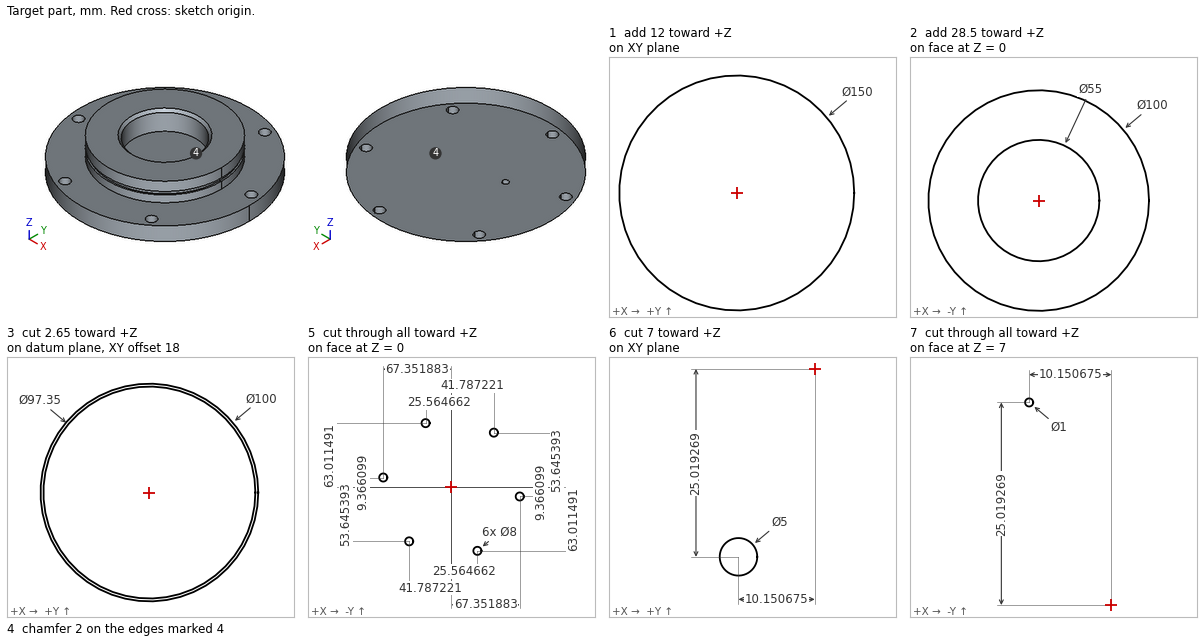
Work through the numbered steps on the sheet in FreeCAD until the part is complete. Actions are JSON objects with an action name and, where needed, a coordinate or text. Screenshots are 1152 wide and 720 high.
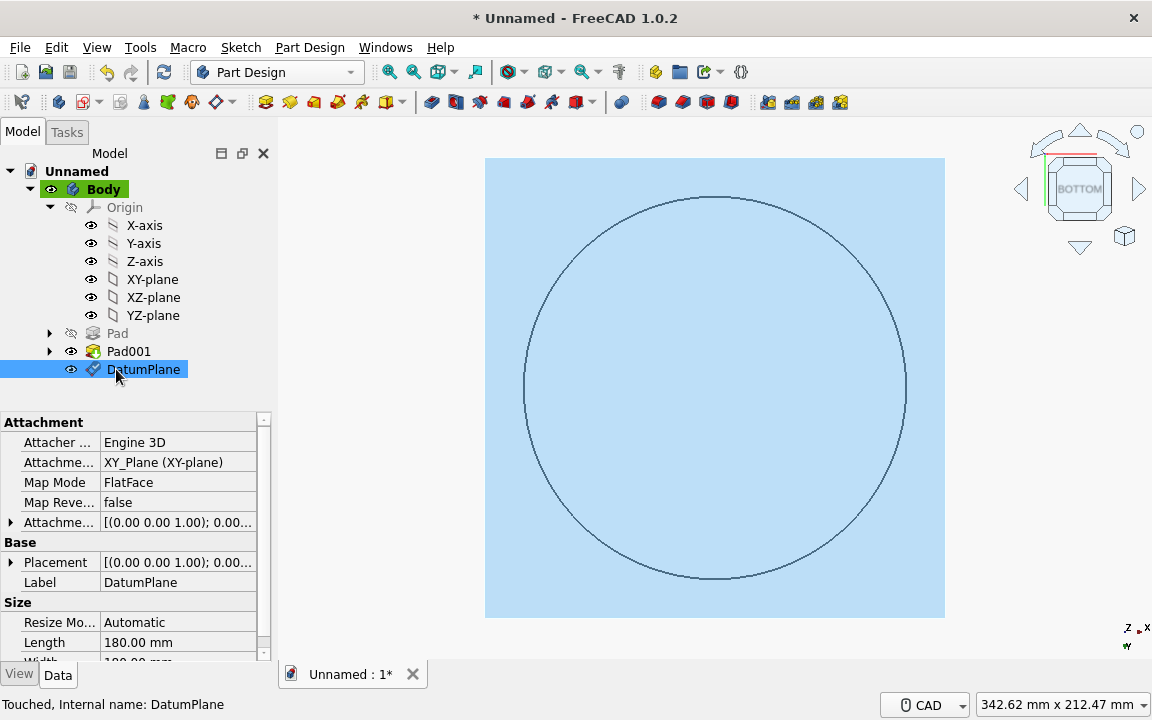
{"action": "left_click", "coordinate": [84, 102]}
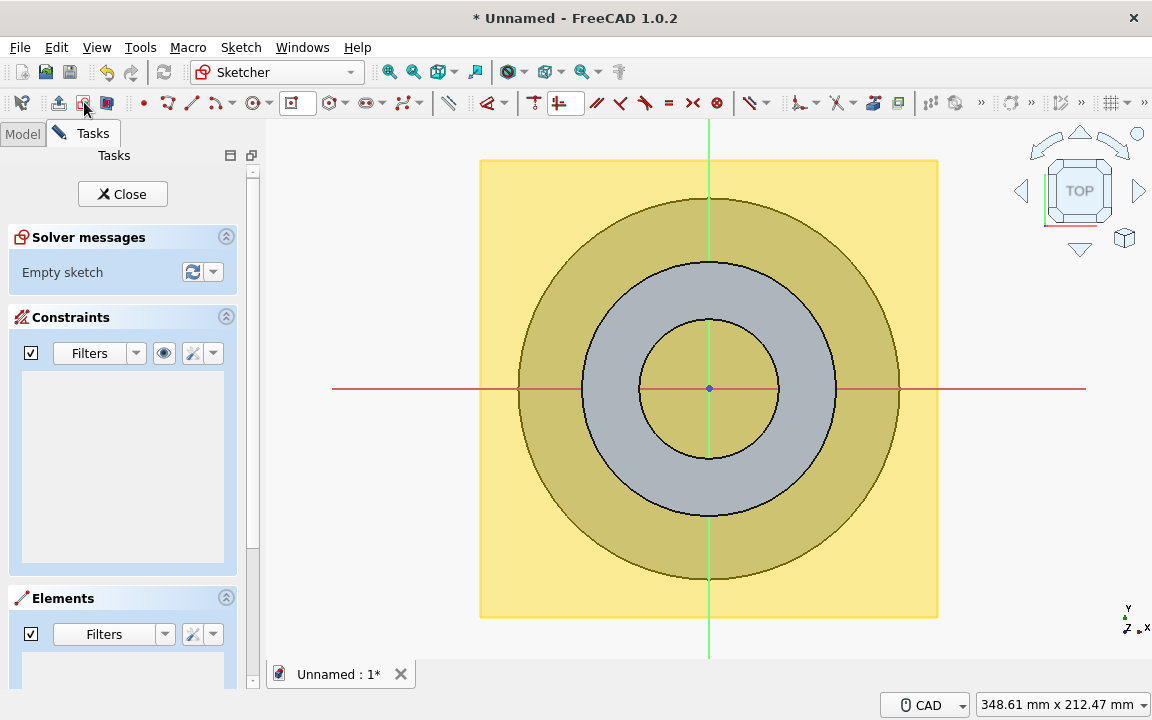
{"action": "key", "text": "q s"}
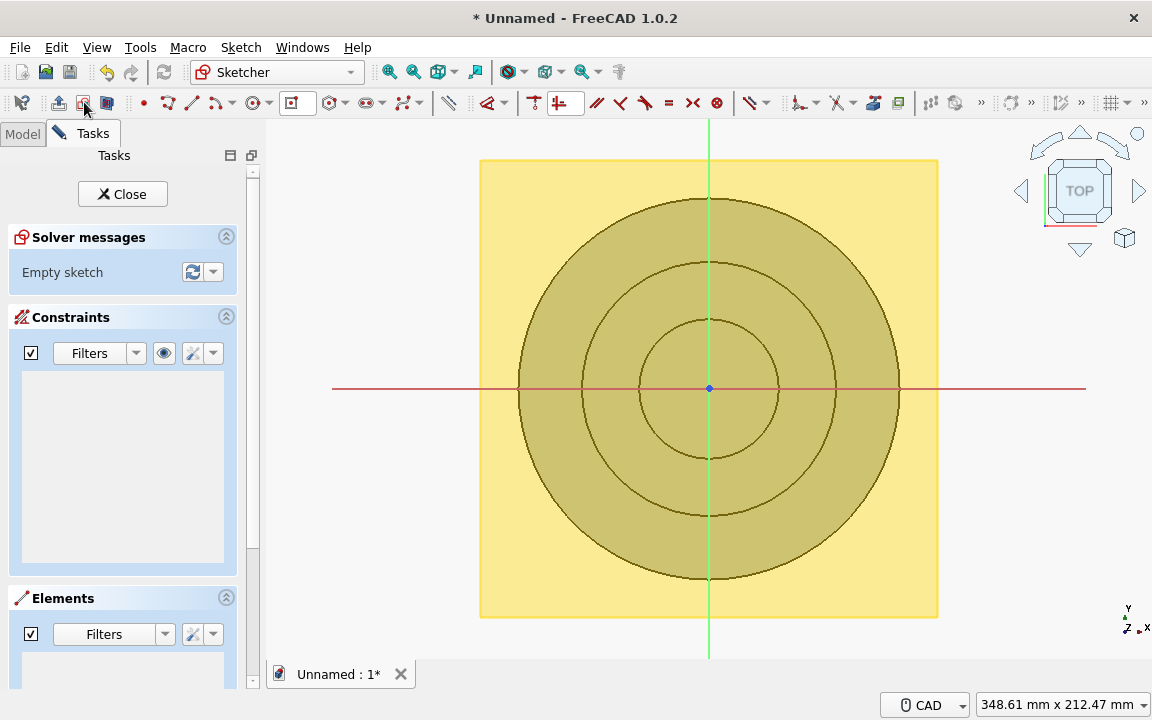
{"action": "left_click", "coordinate": [254, 104]}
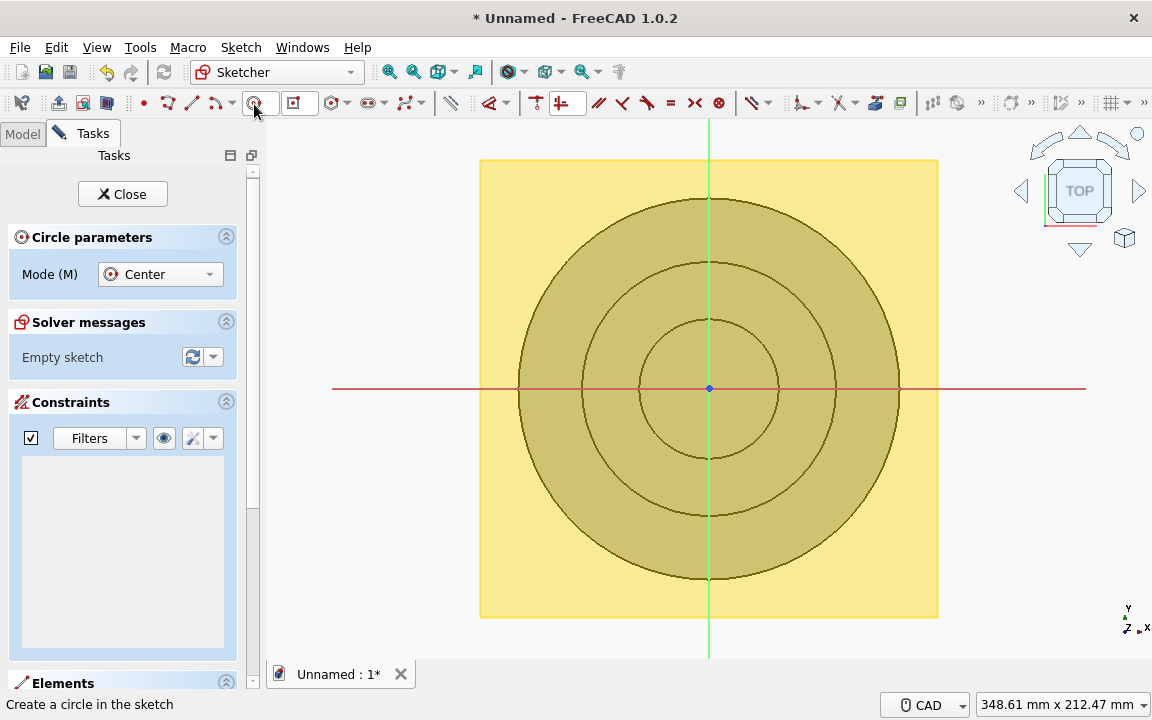
{"action": "left_click", "coordinate": [709, 389]}
{"action": "mouse_move", "coordinate": [799, 299]}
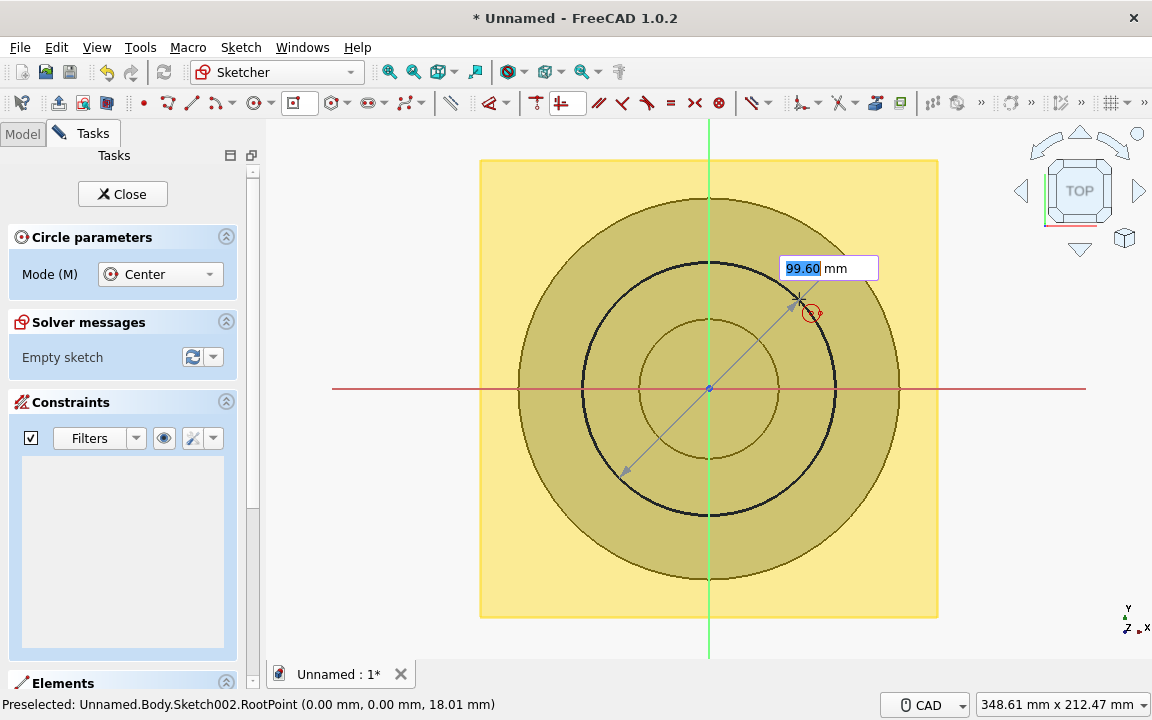
{"action": "type", "text": "100"}
{"action": "key", "text": "Return"}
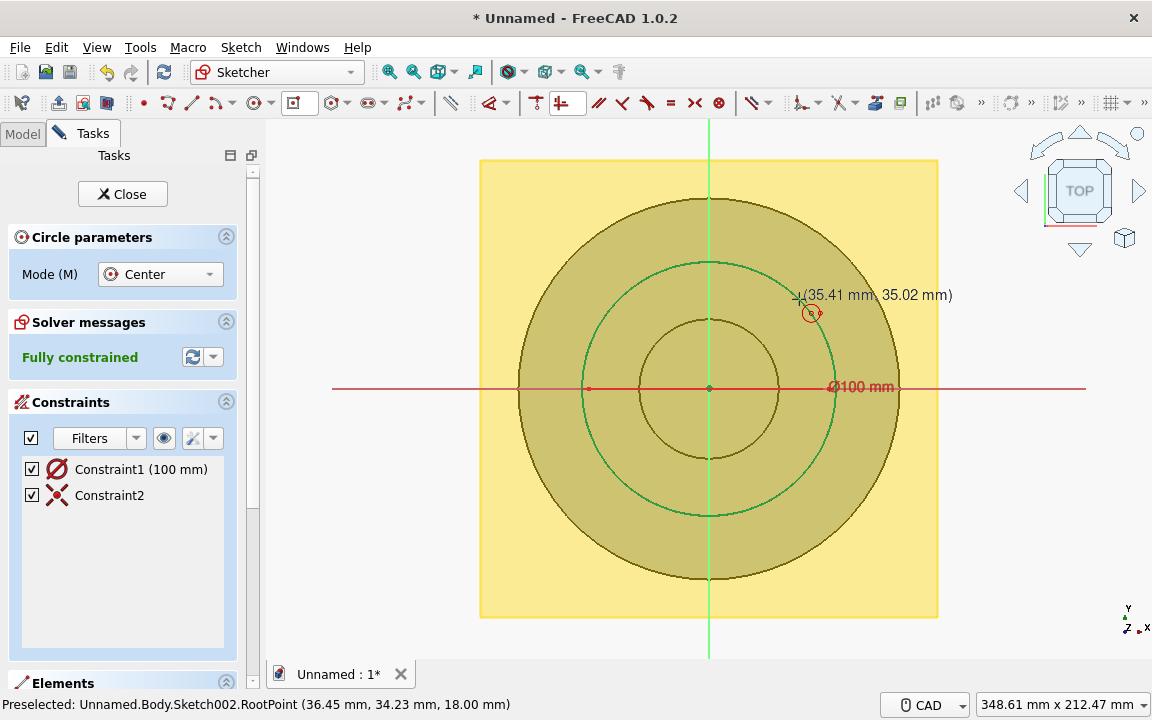
{"action": "left_click", "coordinate": [709, 389]}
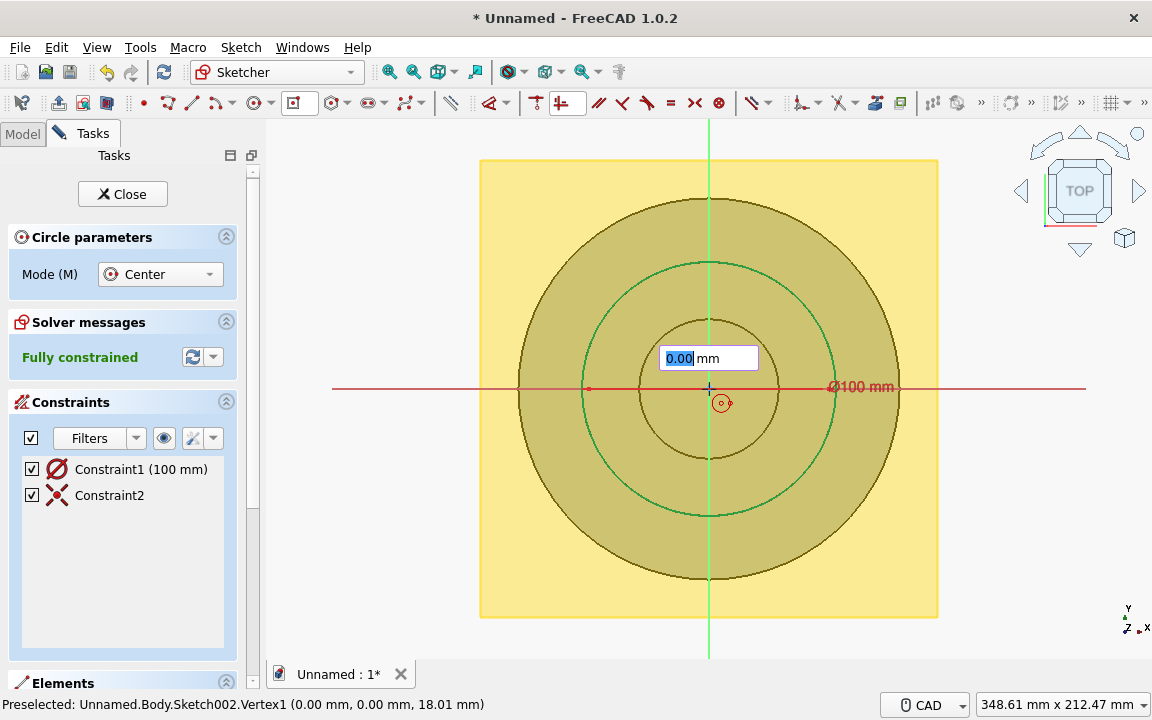
{"action": "scroll", "coordinate": [796, 476], "scroll_direction": "up", "scroll_amount": 8}
{"action": "mouse_move", "coordinate": [796, 476]}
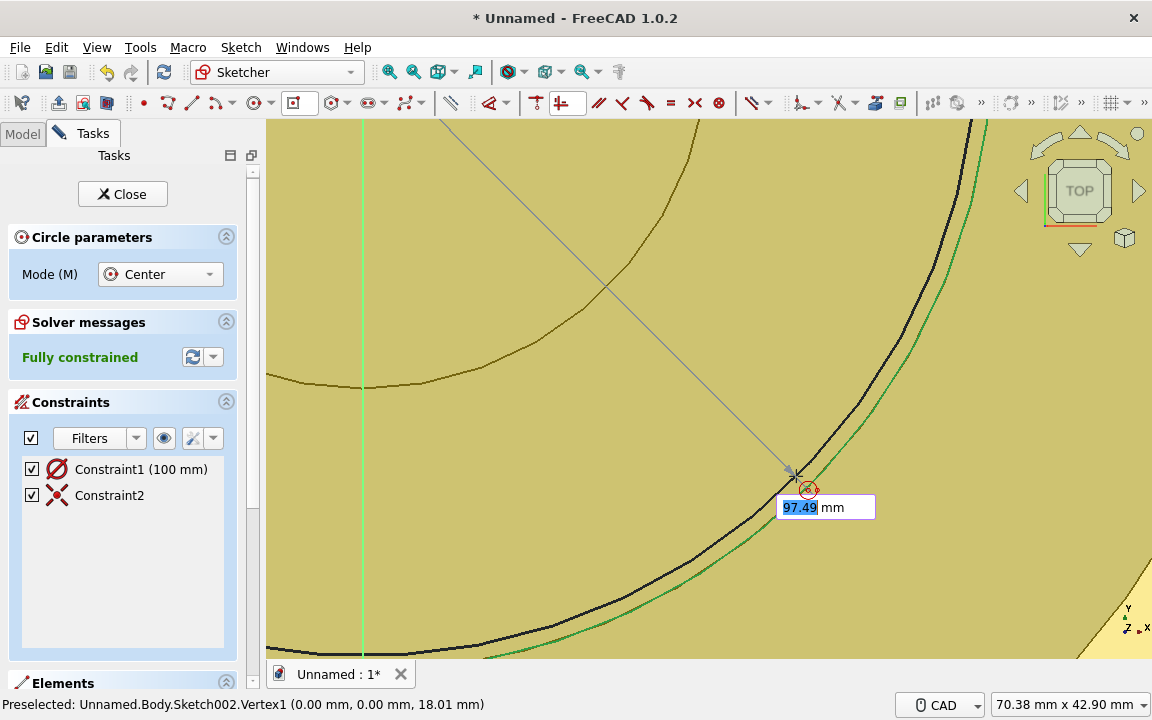
{"action": "type", "text": "97.35"}
{"action": "key", "text": "Return"}
{"action": "key", "text": "Escape"}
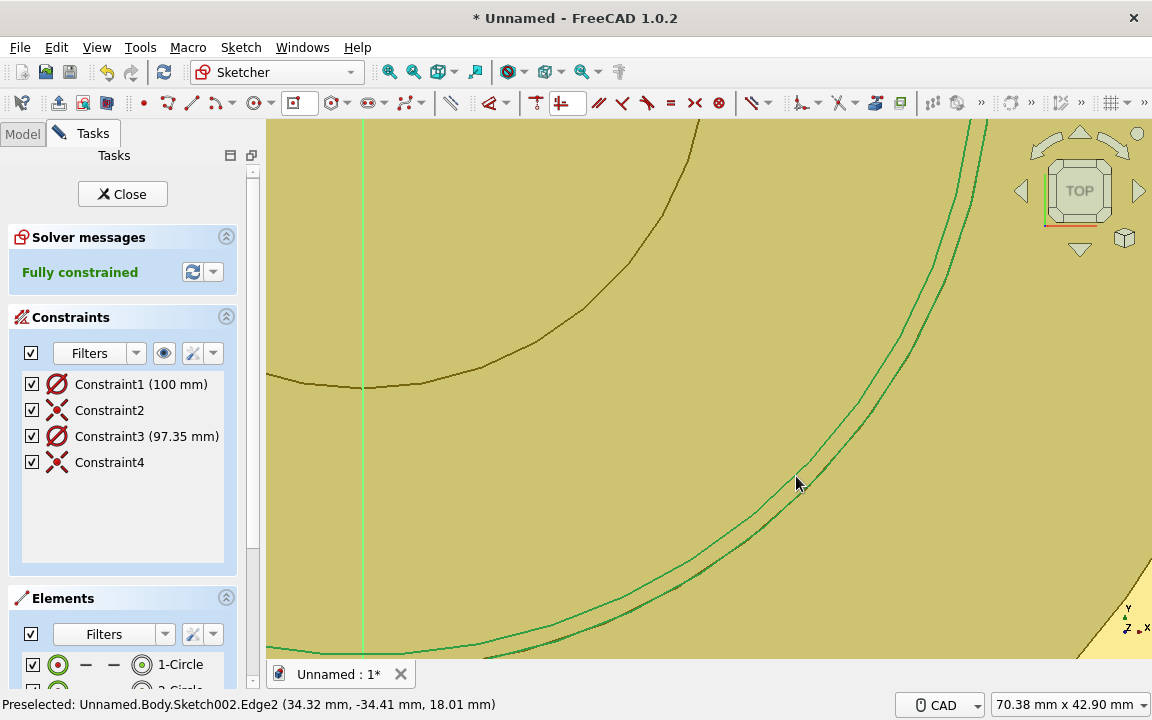
{"action": "left_click", "coordinate": [123, 194]}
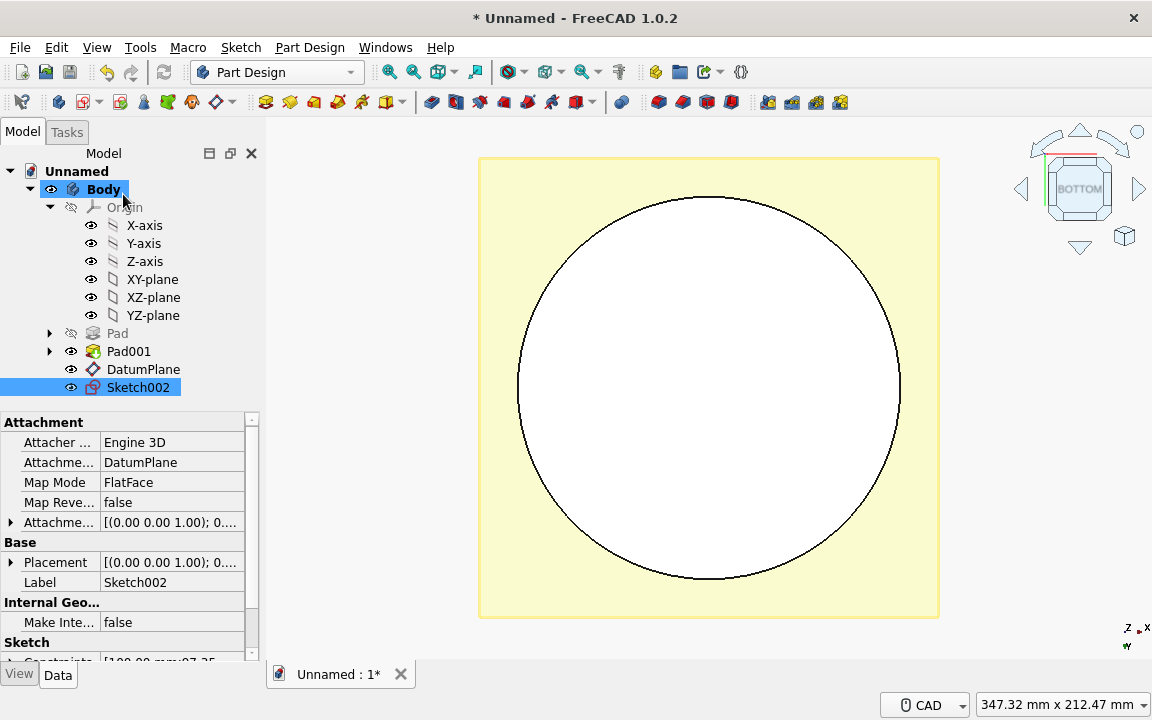
{"action": "left_click", "coordinate": [432, 102]}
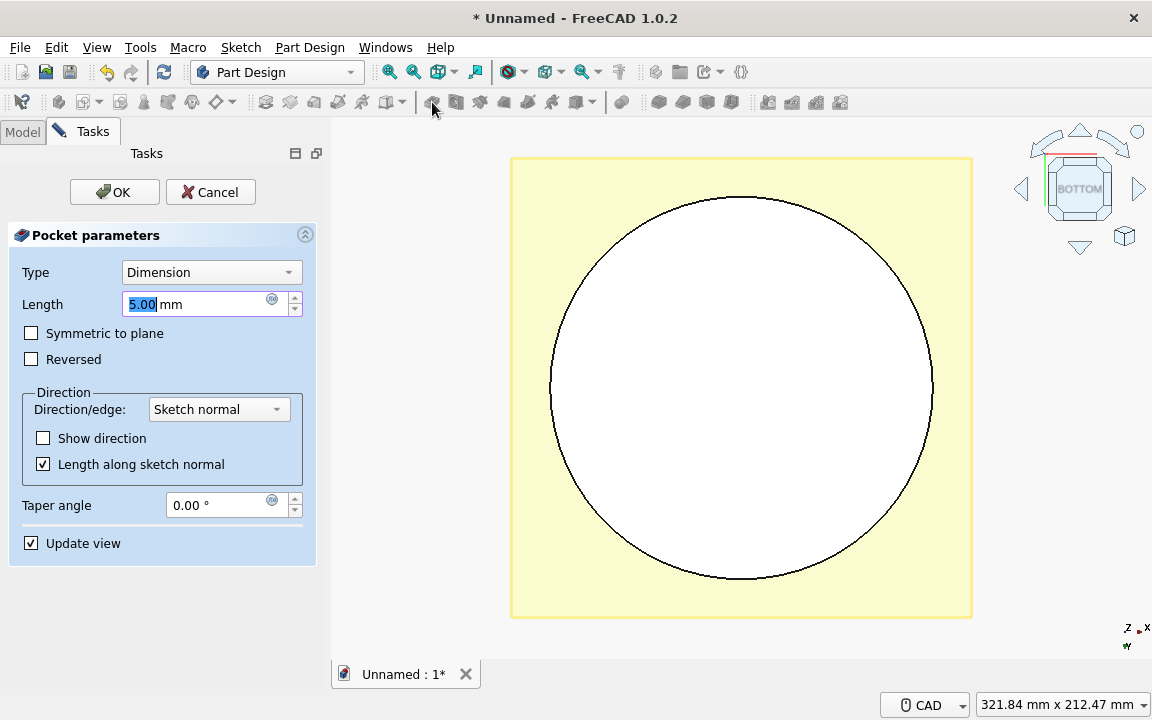
{"action": "type", "text": "2.65"}
{"action": "key", "text": "Tab"}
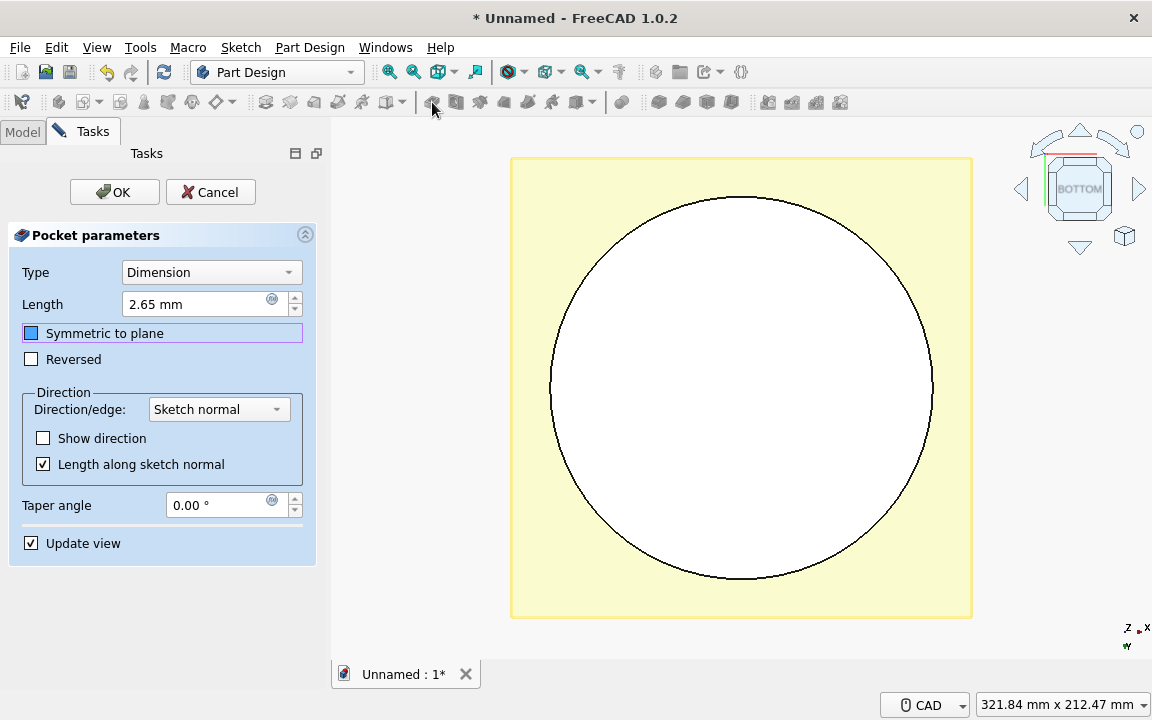
{"action": "left_click", "coordinate": [30, 359]}